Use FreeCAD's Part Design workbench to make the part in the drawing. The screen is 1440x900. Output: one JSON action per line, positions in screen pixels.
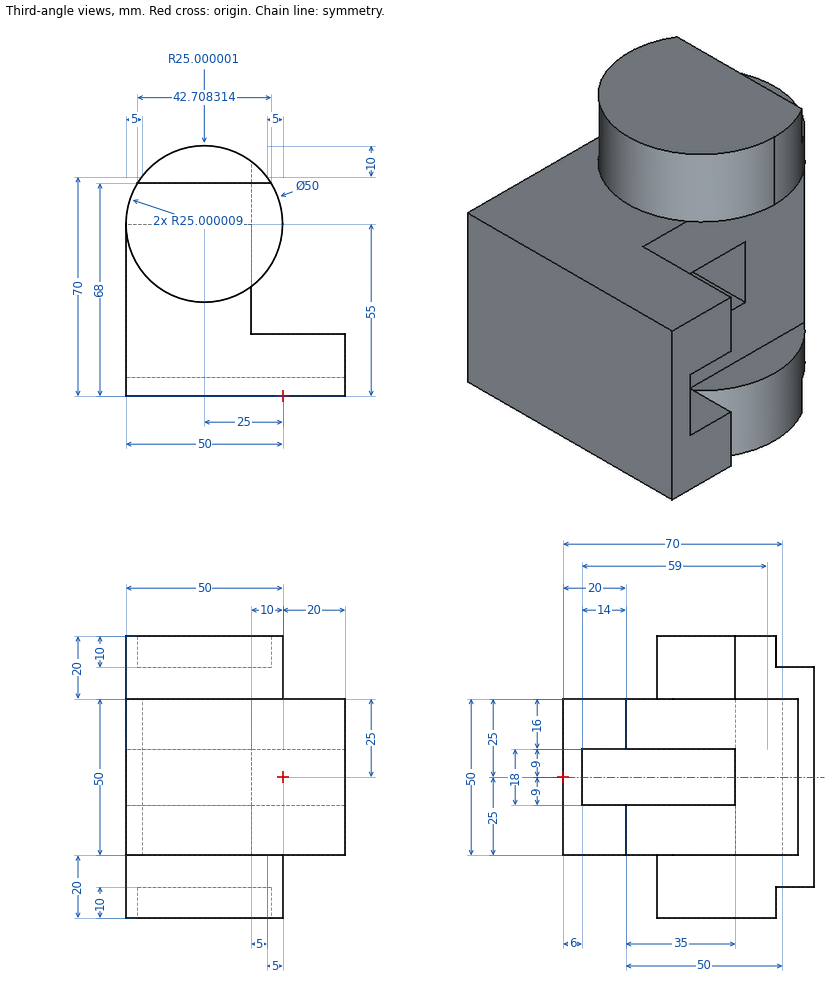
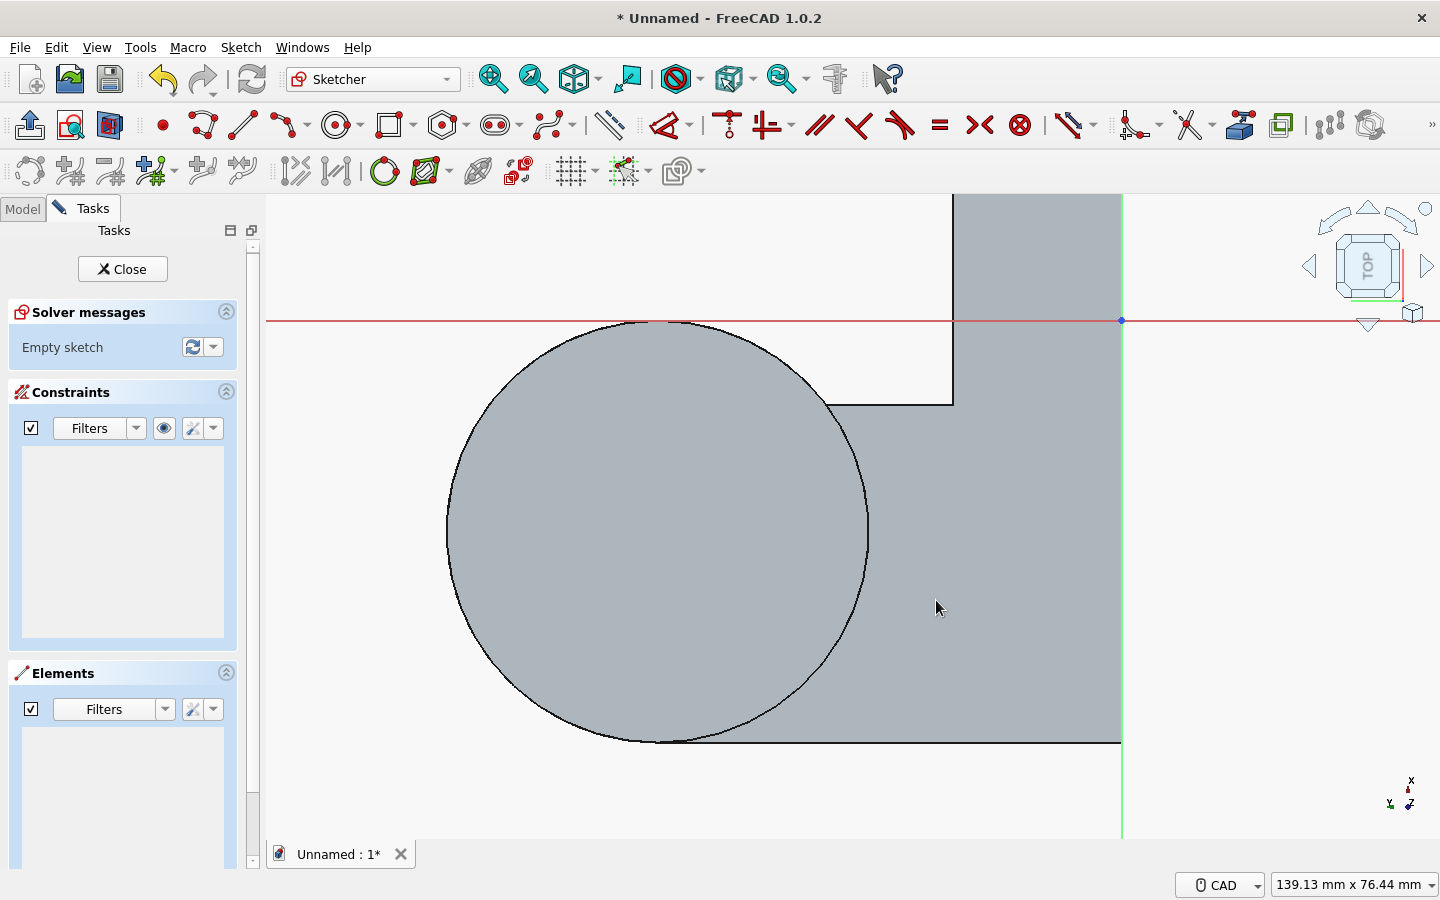
{"action": "left_click", "coordinate": [244, 126]}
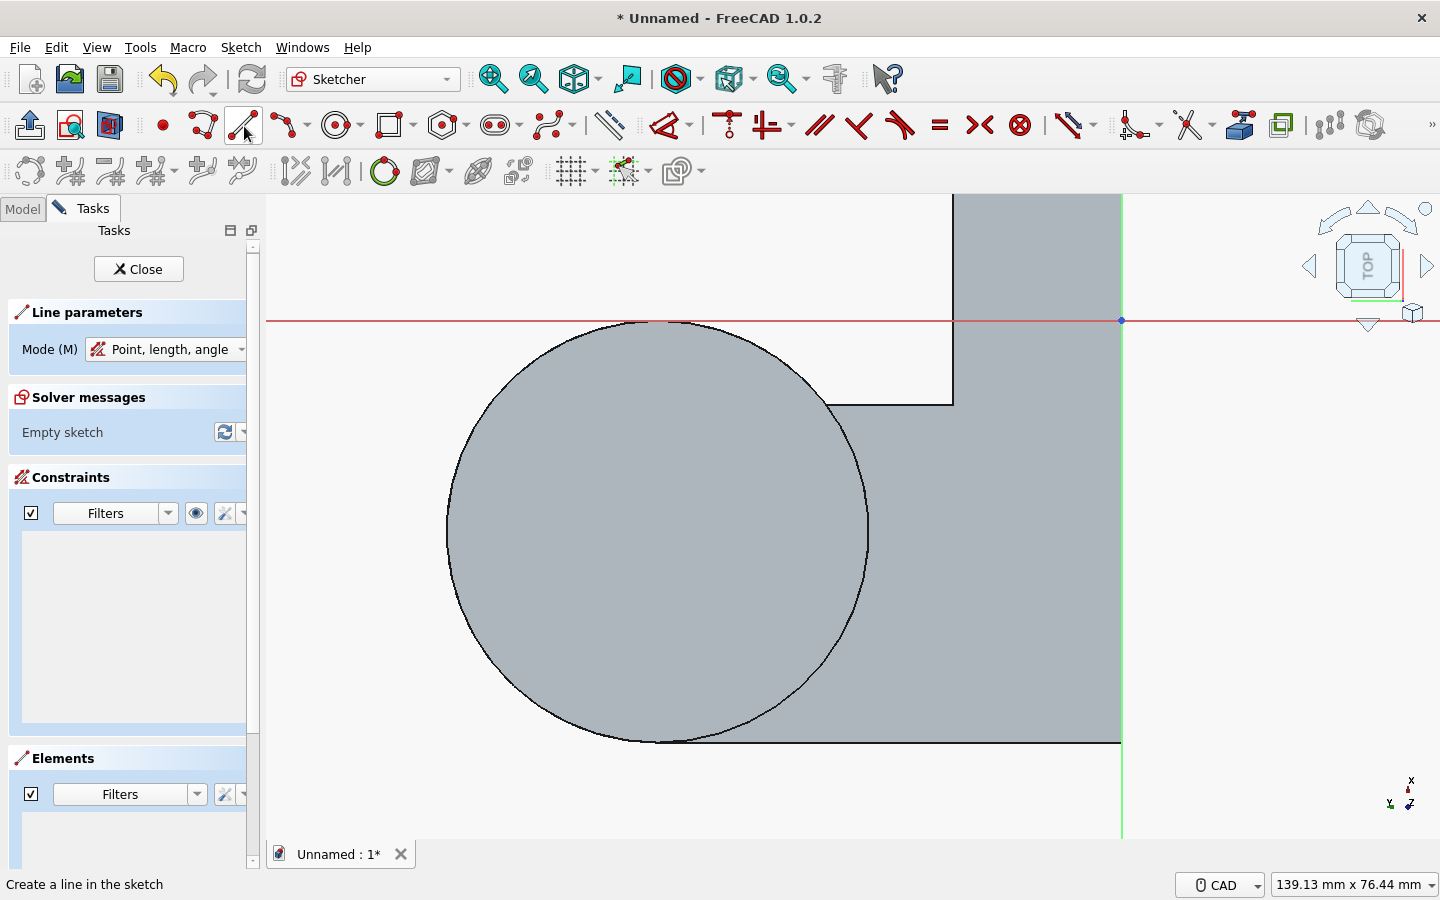
{"action": "left_click", "coordinate": [548, 712]}
{"action": "left_click", "coordinate": [548, 352]}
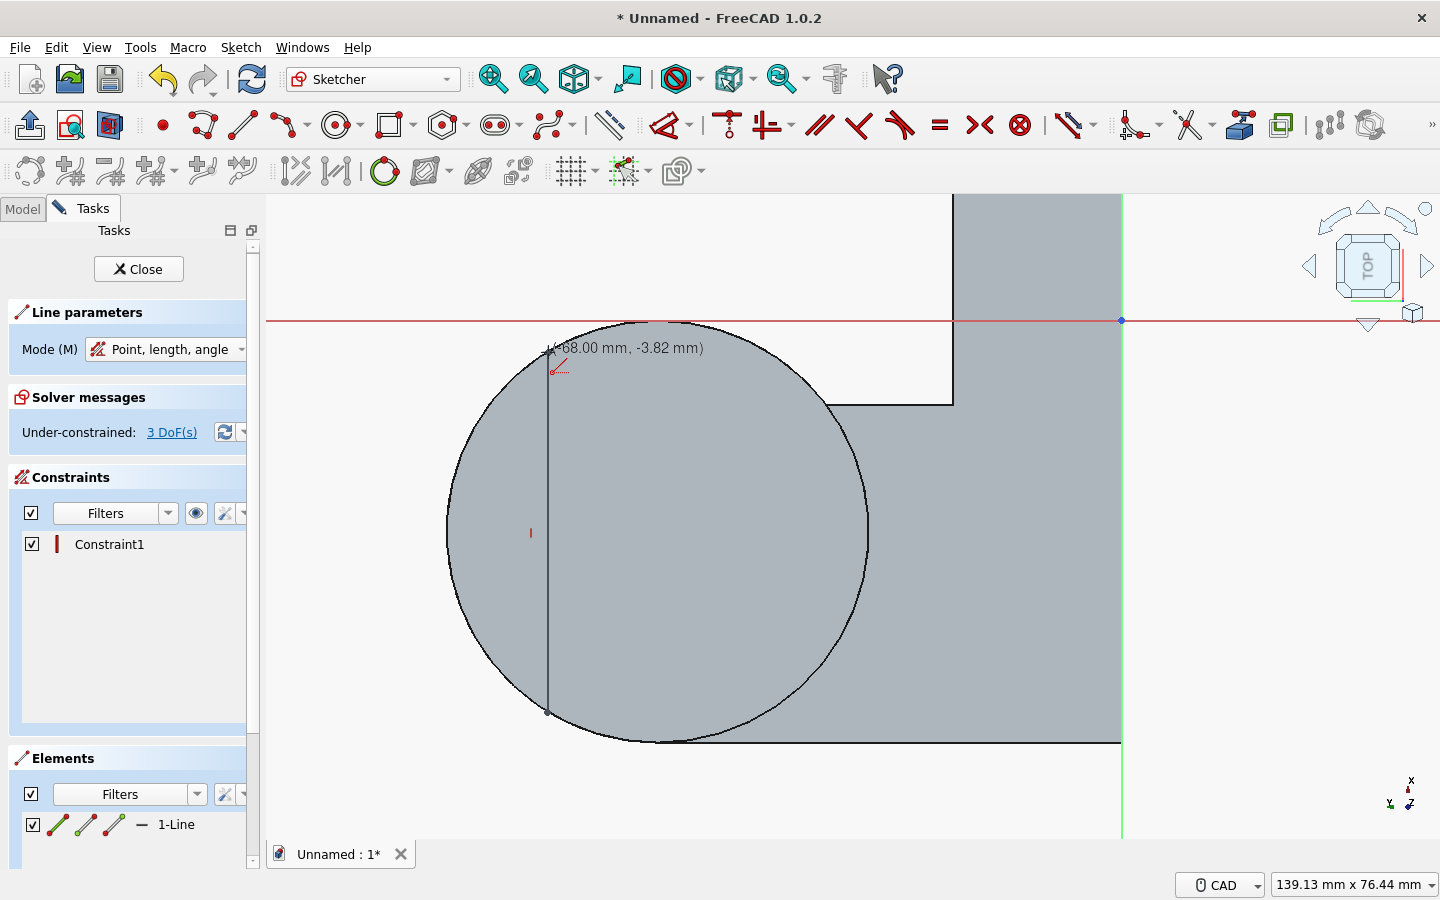
{"action": "left_click", "coordinate": [284, 126]}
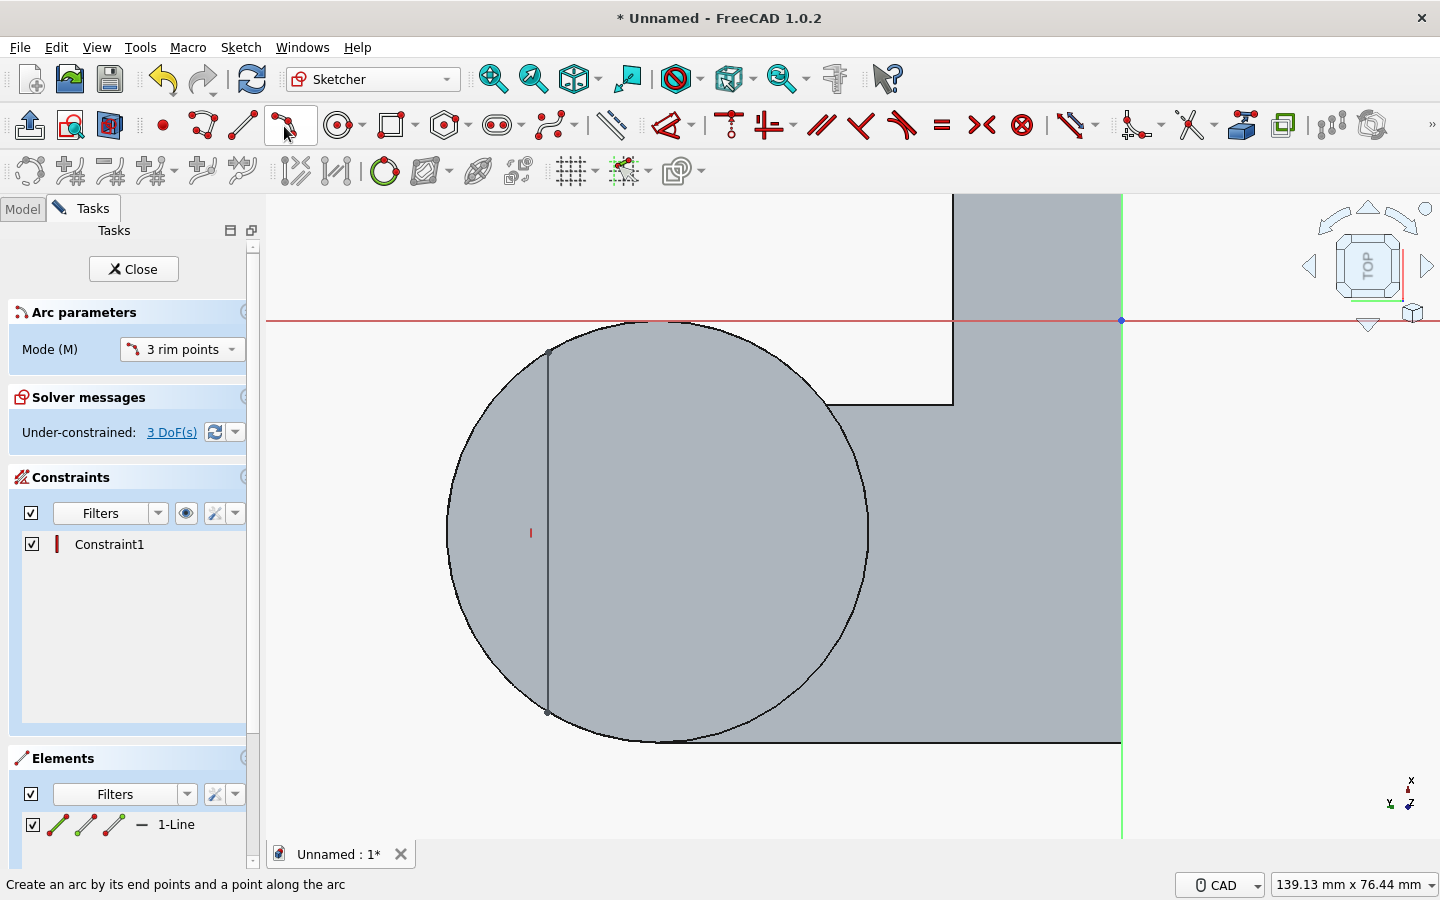
{"action": "left_click", "coordinate": [548, 353]}
{"action": "left_click", "coordinate": [548, 713]}
{"action": "left_click", "coordinate": [447, 532]}
{"action": "key", "text": "Escape"}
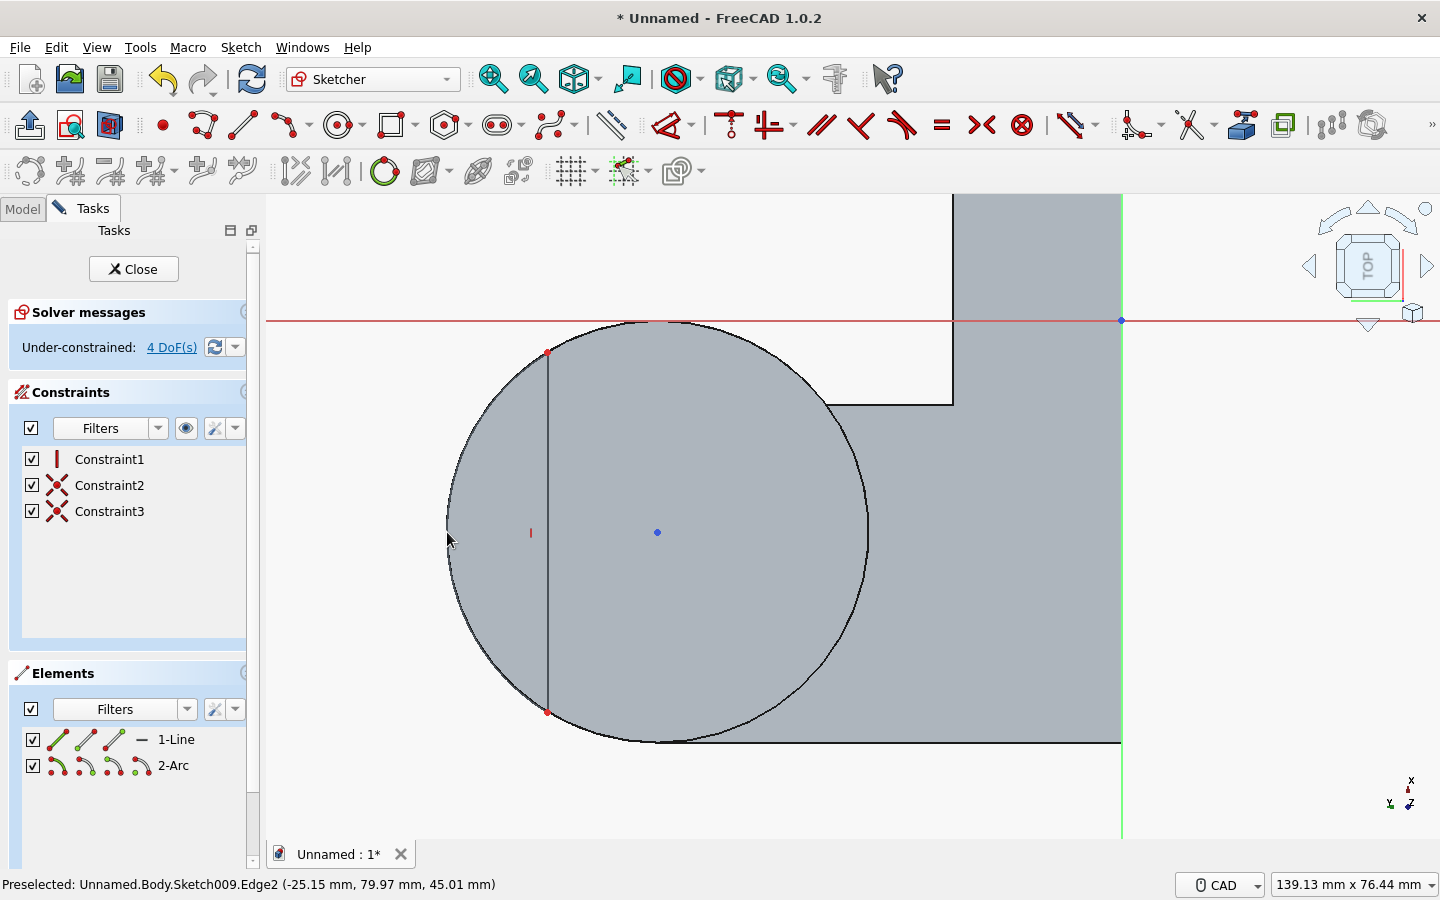
{"action": "left_click", "coordinate": [666, 126]}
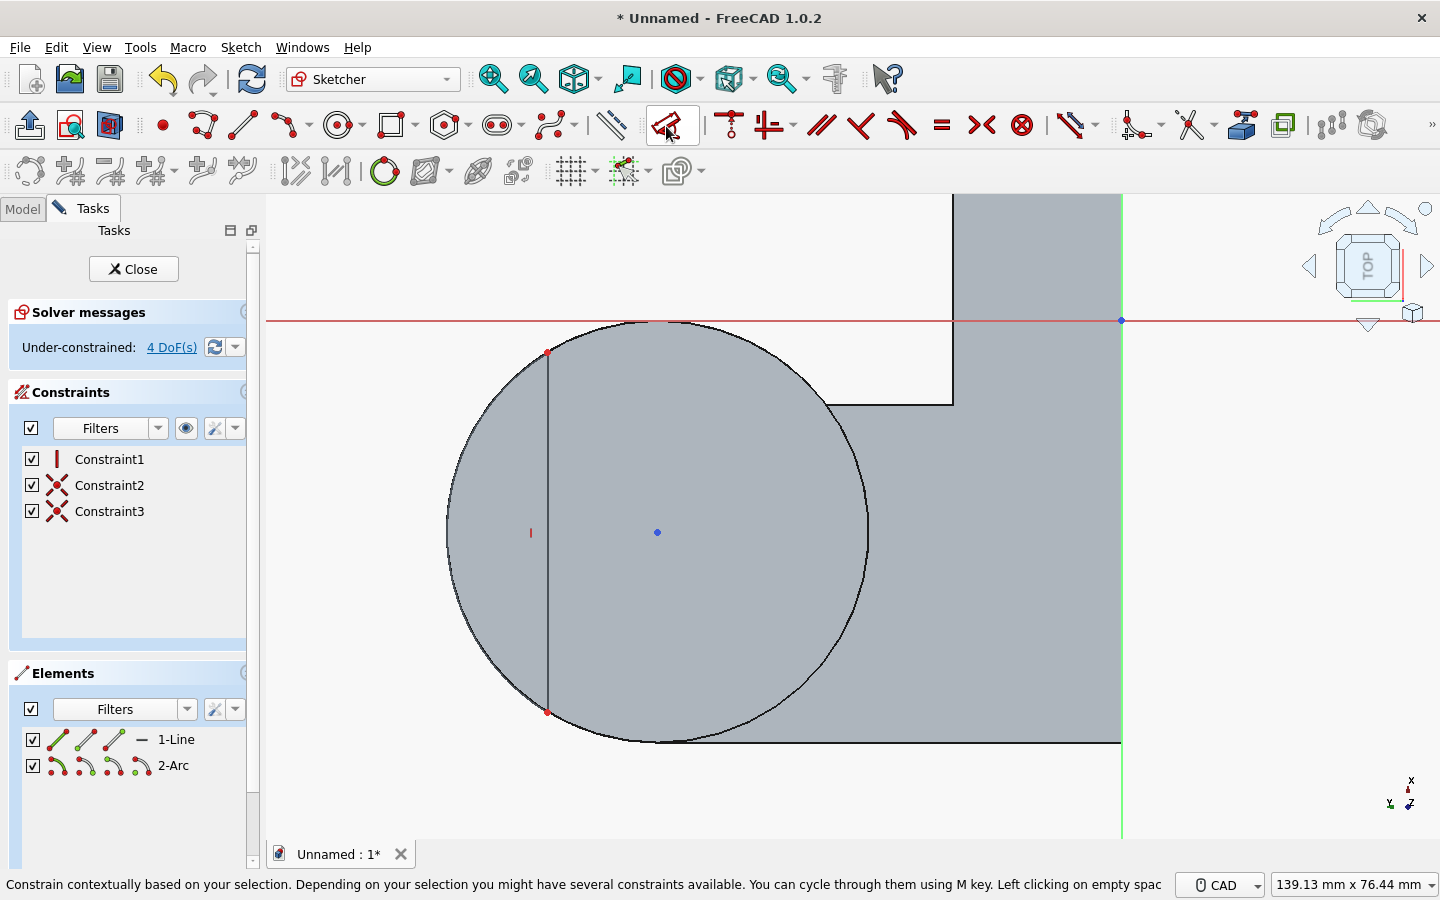
{"action": "left_click", "coordinate": [464, 449]}
{"action": "left_click", "coordinate": [435, 436]}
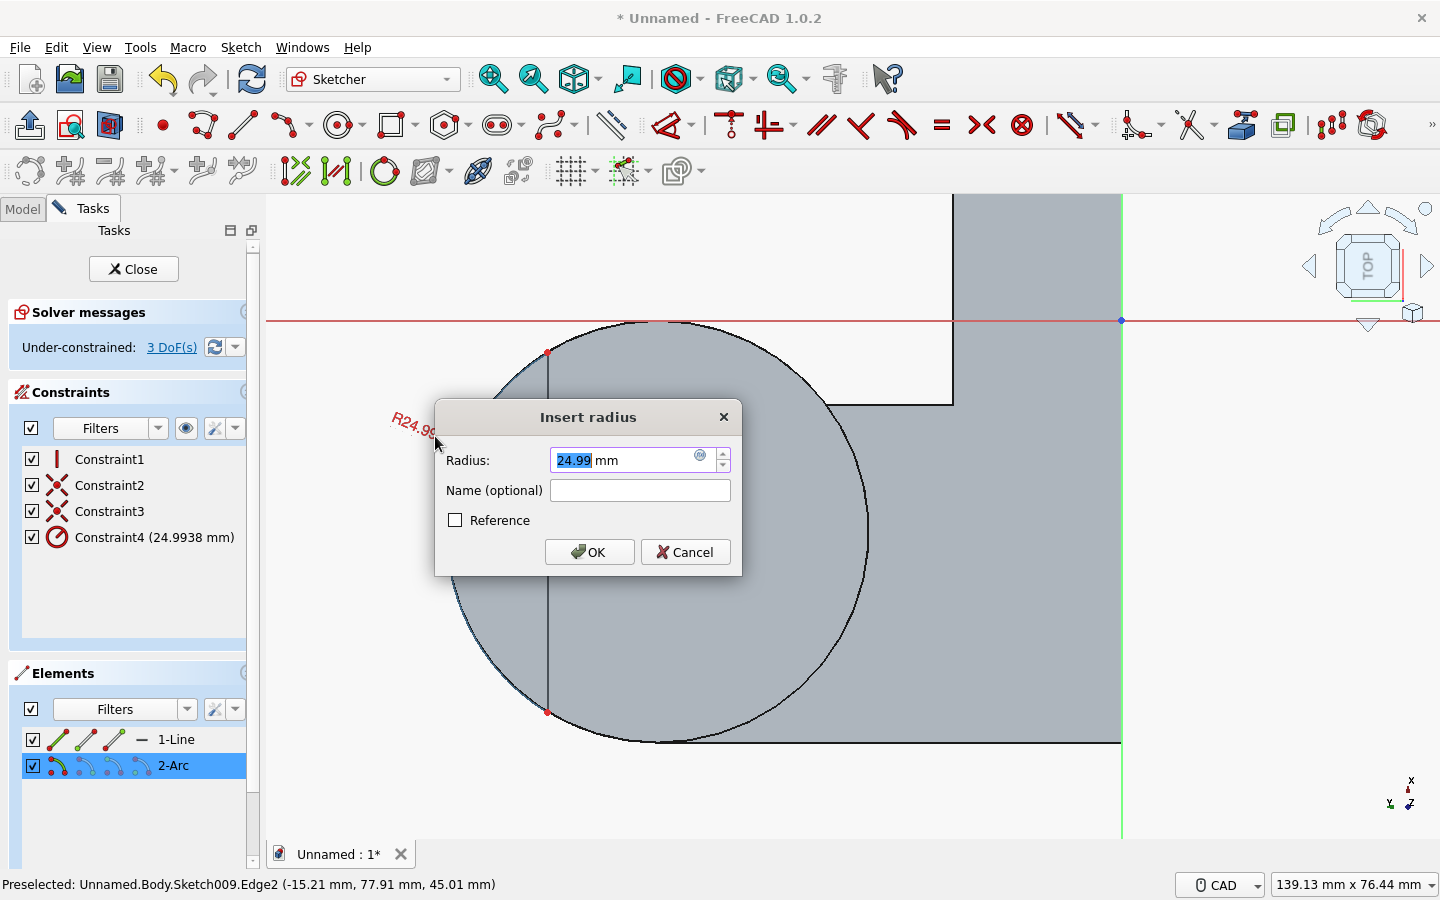
{"action": "type", "text": "25.000001"}
{"action": "key", "text": "Return"}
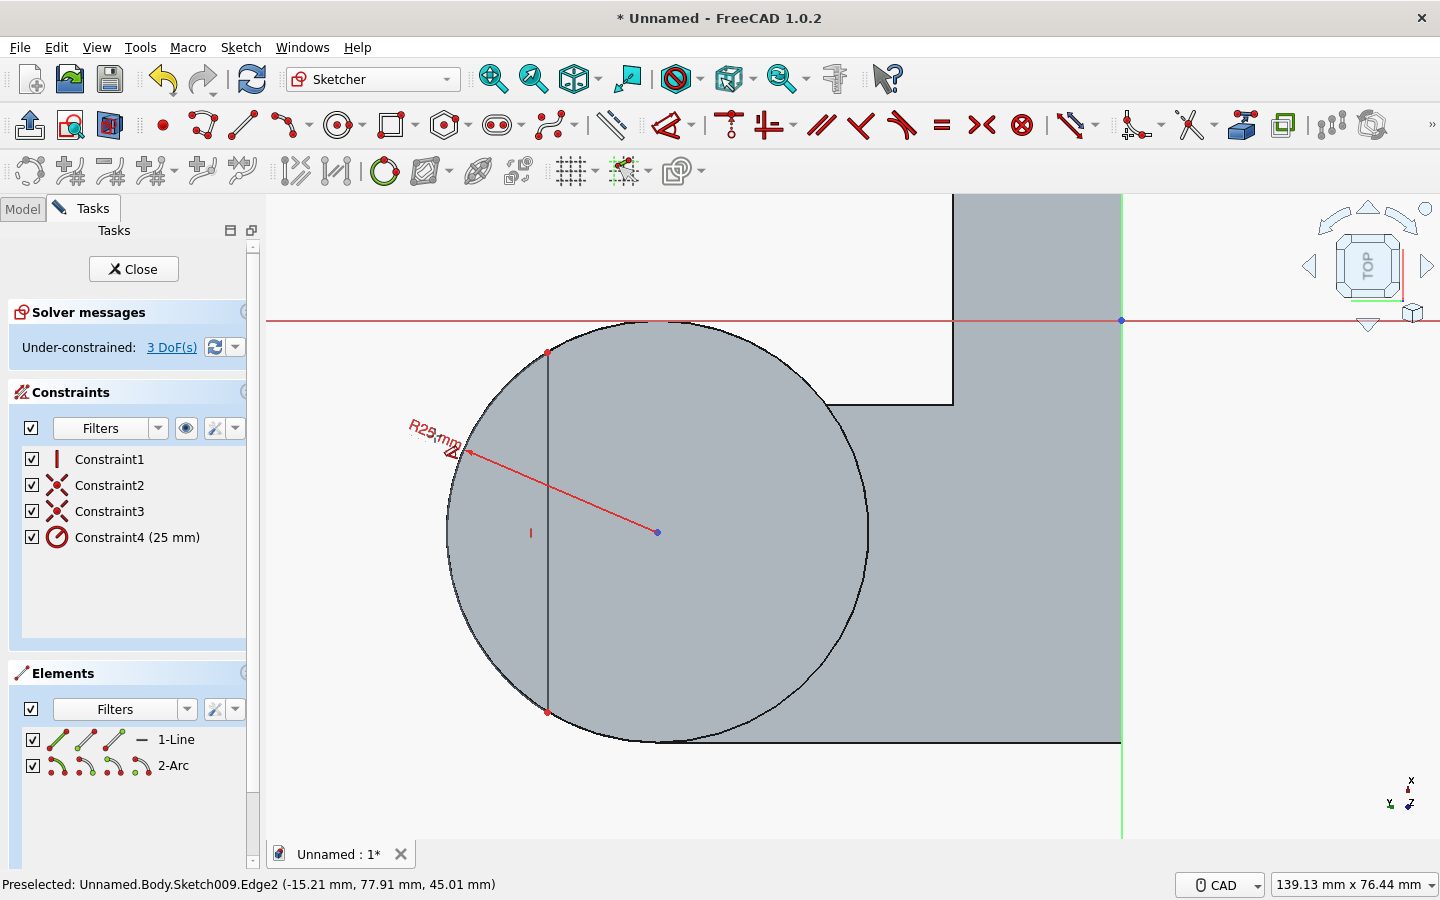
{"action": "left_click", "coordinate": [548, 713]}
{"action": "left_click", "coordinate": [835, 747]}